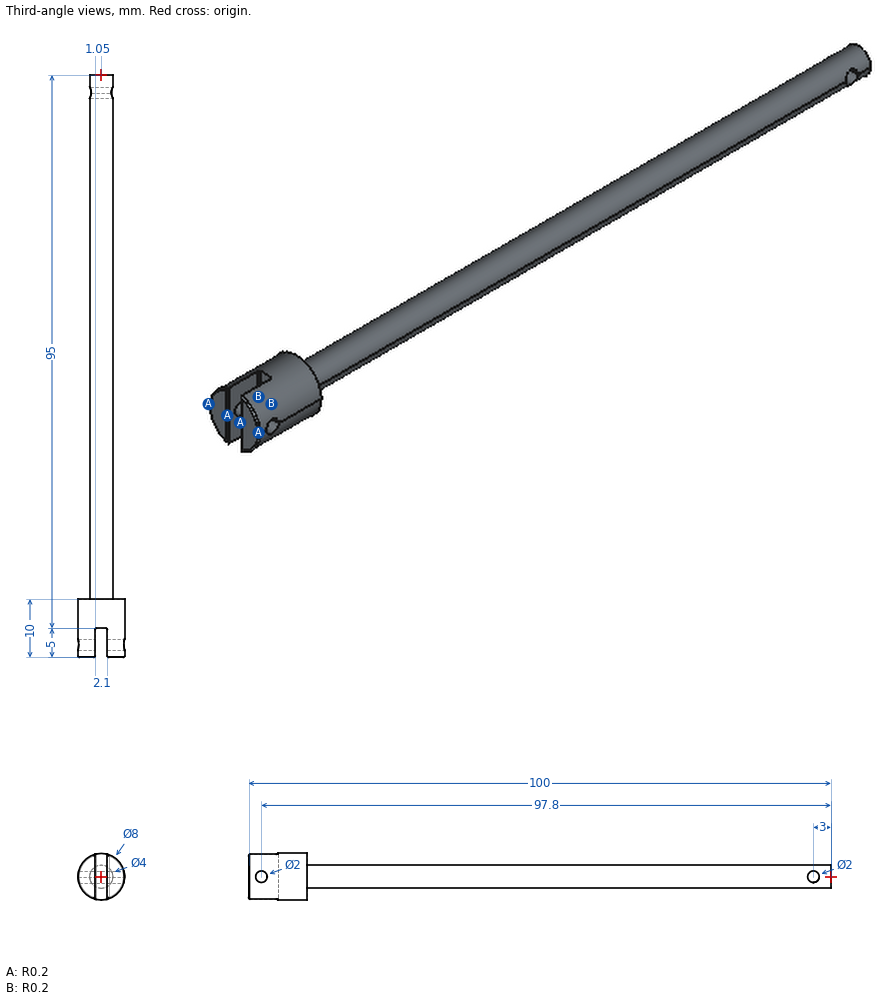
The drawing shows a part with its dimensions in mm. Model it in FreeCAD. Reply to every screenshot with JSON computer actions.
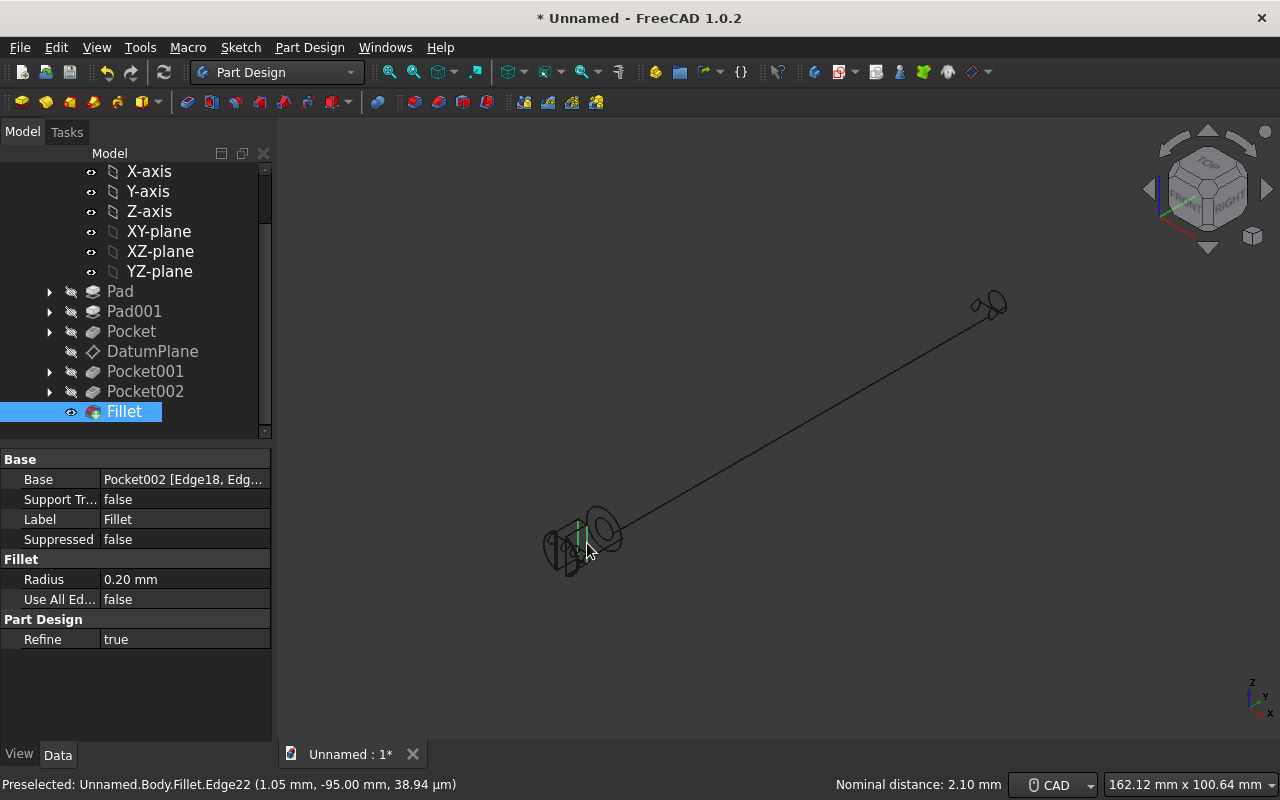
{"action": "key", "text": "v 1"}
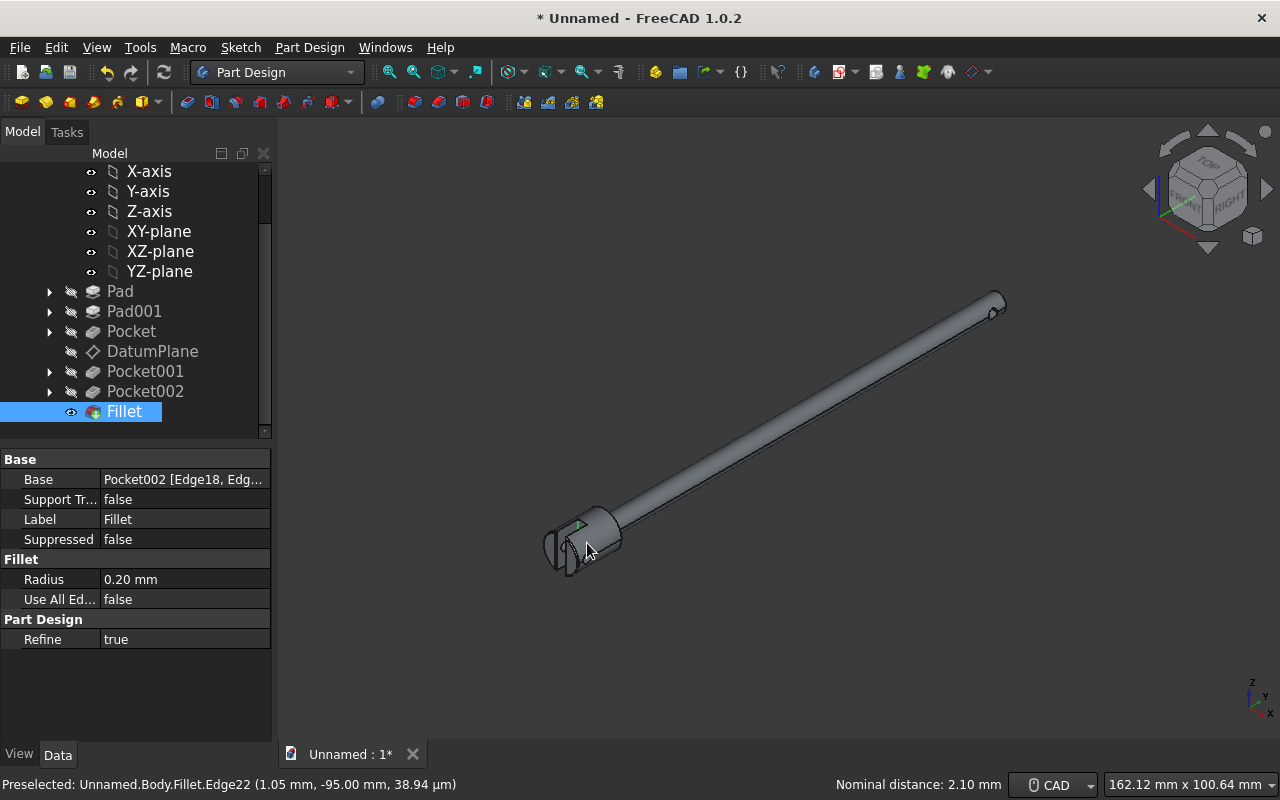
{"action": "left_click", "coordinate": [416, 102]}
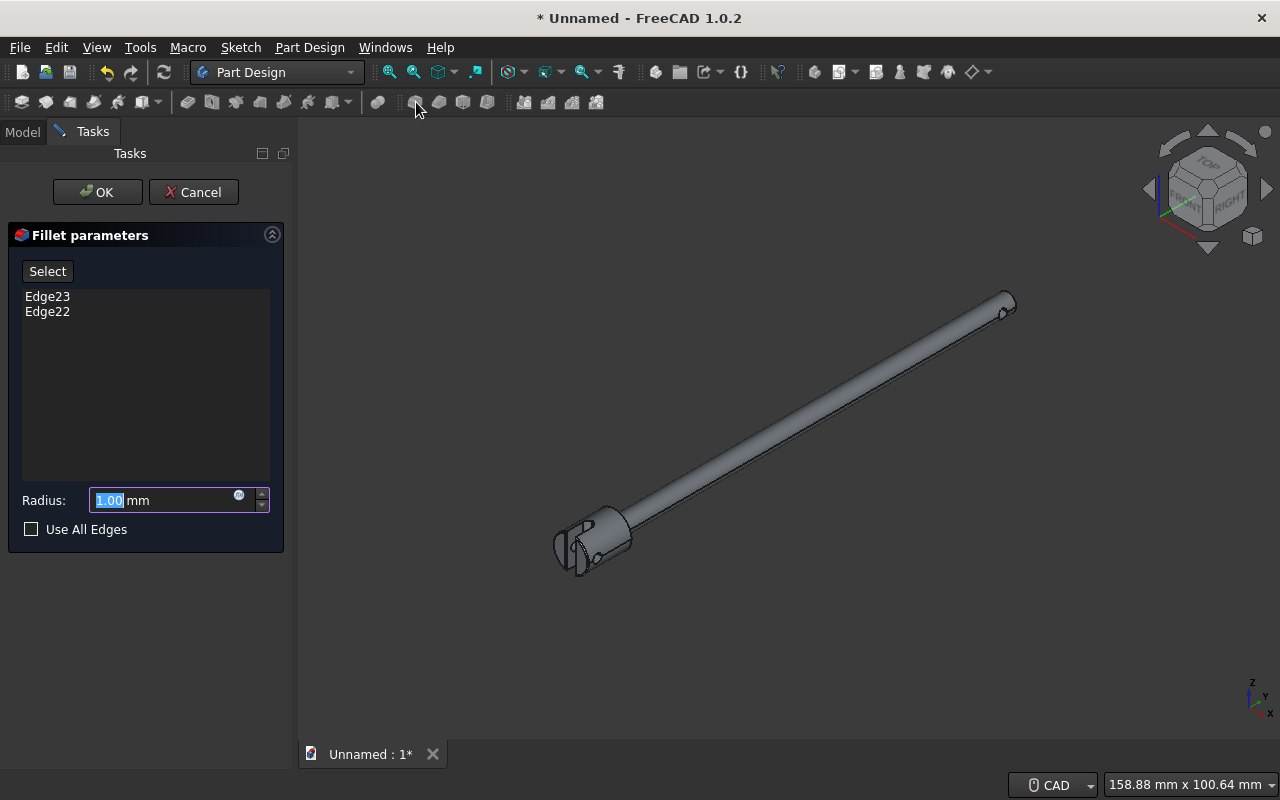
{"action": "type", "text": "0.2"}
{"action": "key", "text": "Tab"}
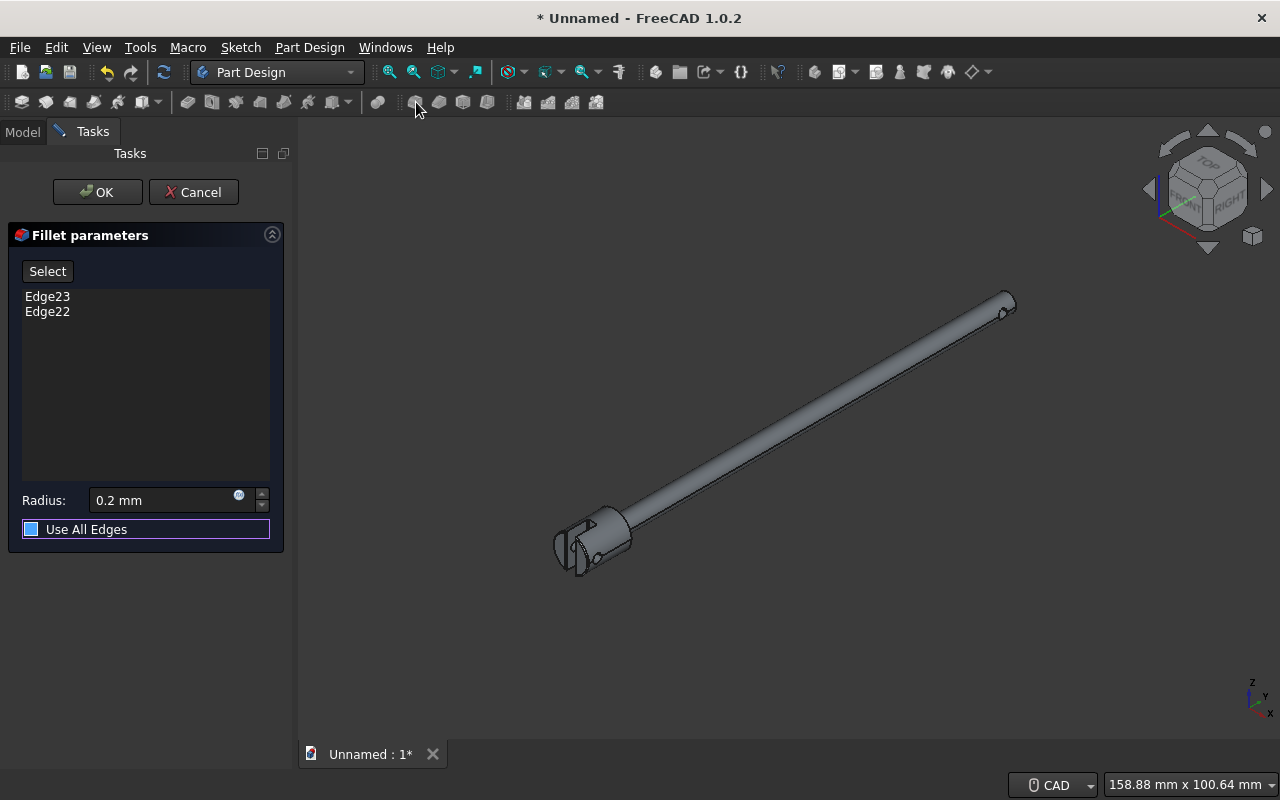
{"action": "left_click", "coordinate": [98, 192]}